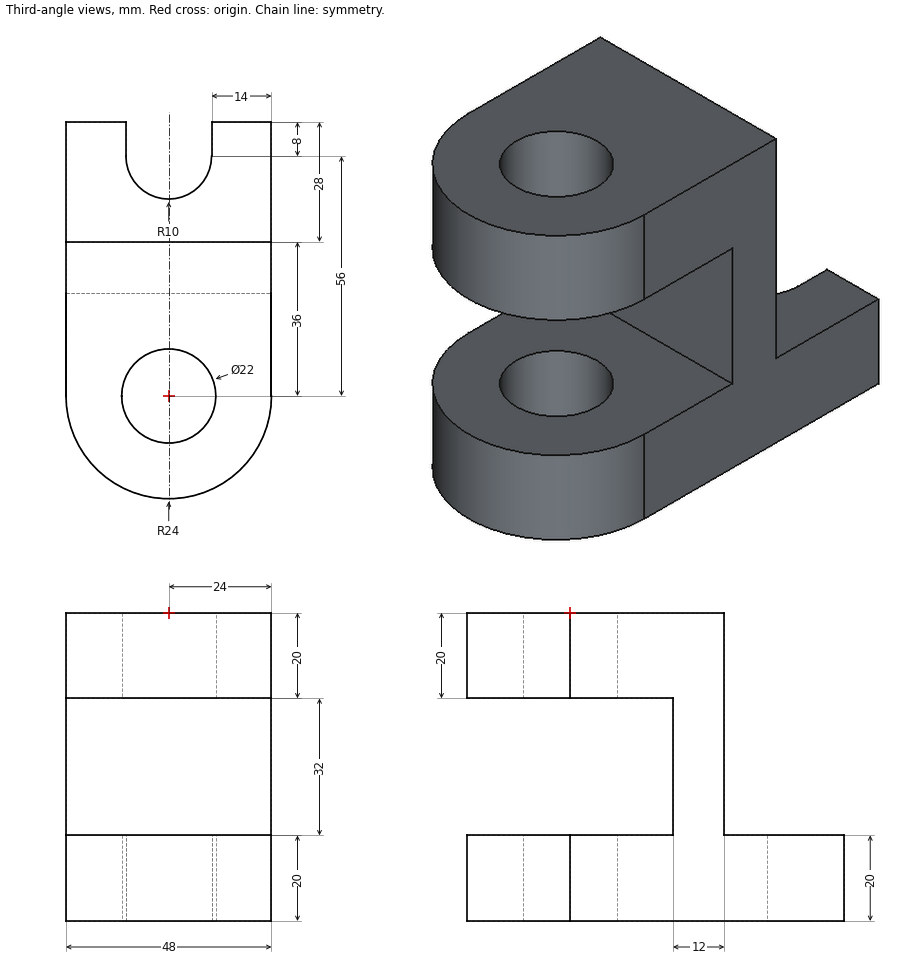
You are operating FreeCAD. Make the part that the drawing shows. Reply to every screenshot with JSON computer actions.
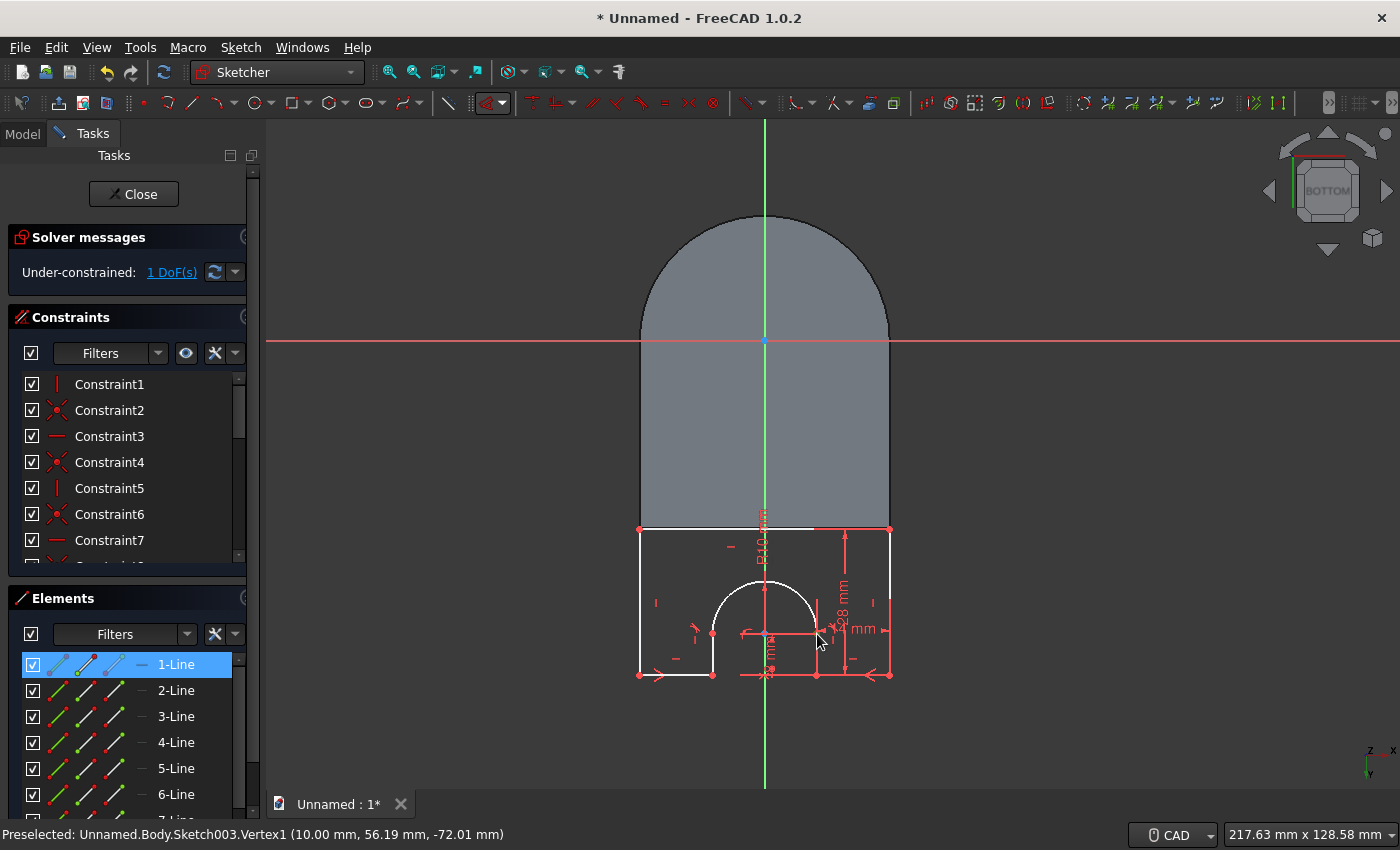
{"action": "key", "text": "i"}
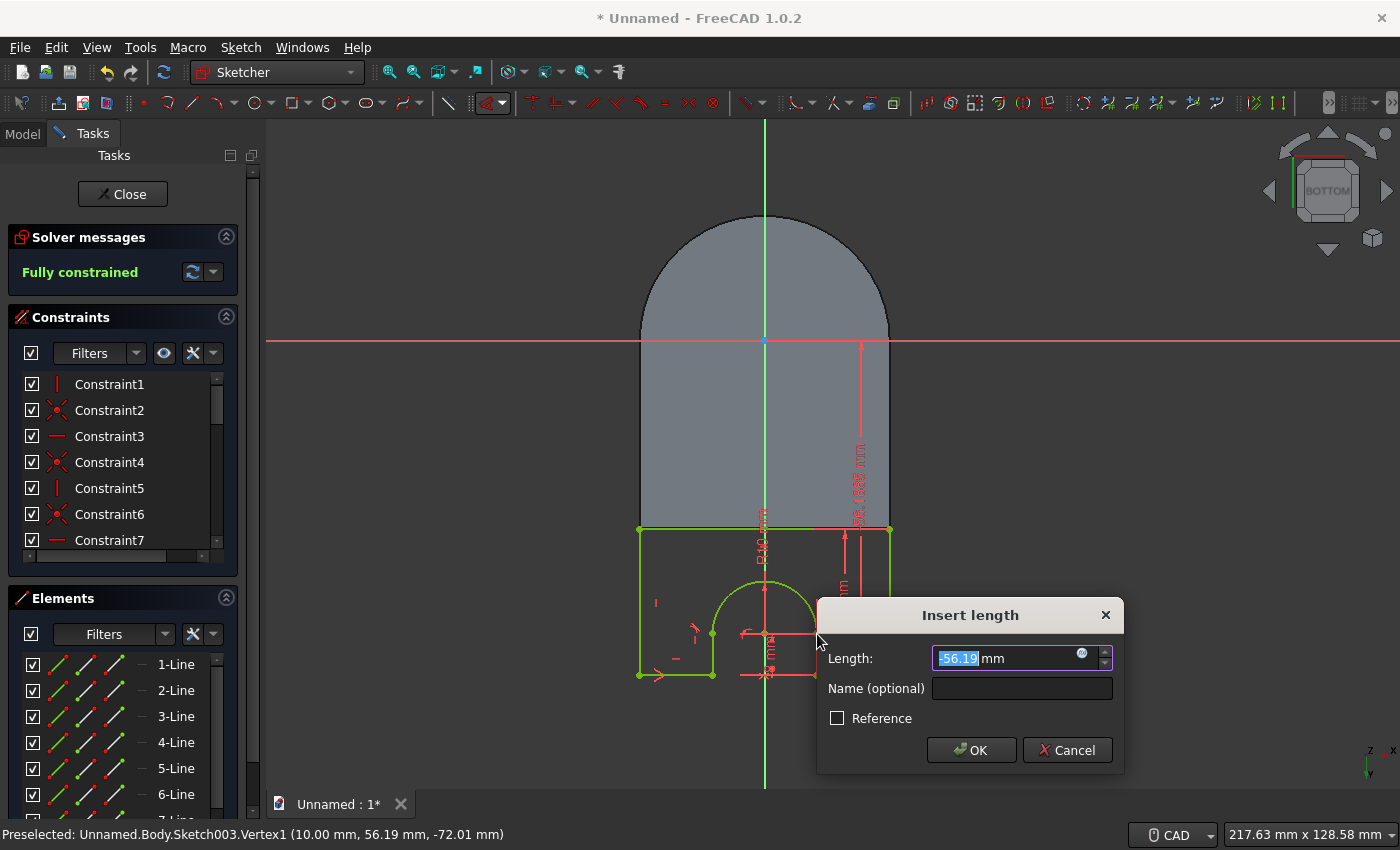
{"action": "type", "text": "-56"}
{"action": "key", "text": "Return"}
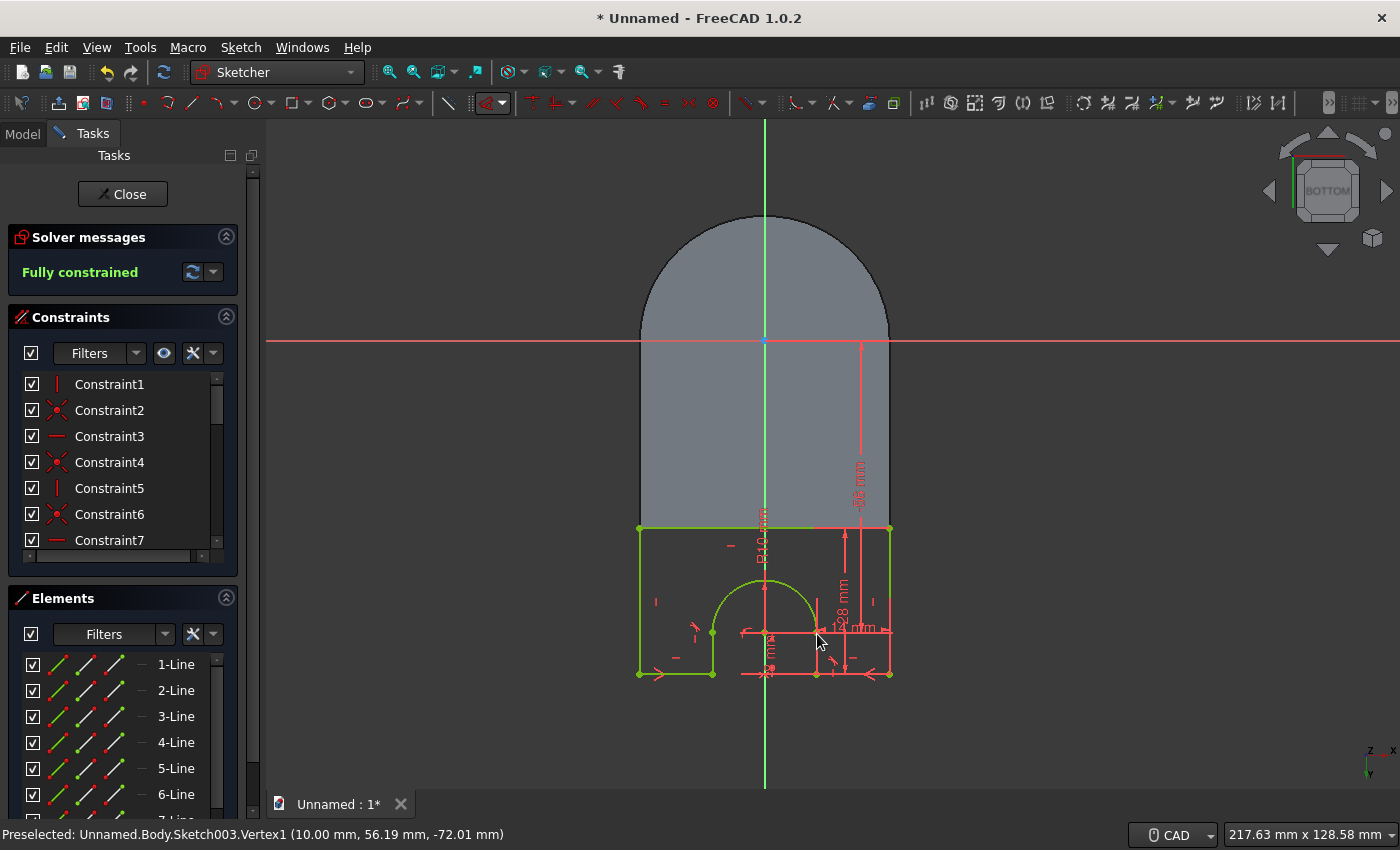
{"action": "left_click", "coordinate": [123, 194]}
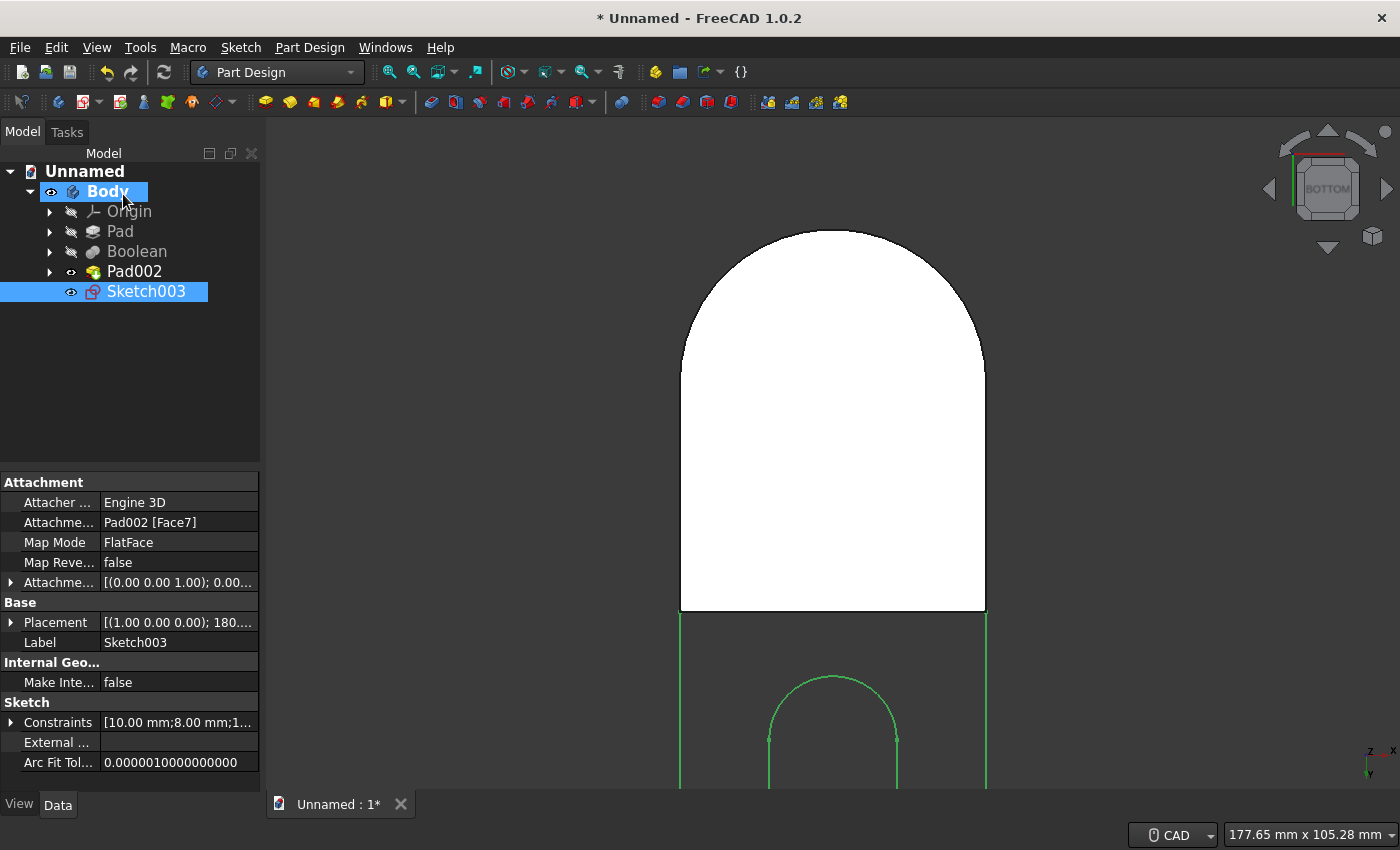
{"action": "left_click", "coordinate": [266, 102]}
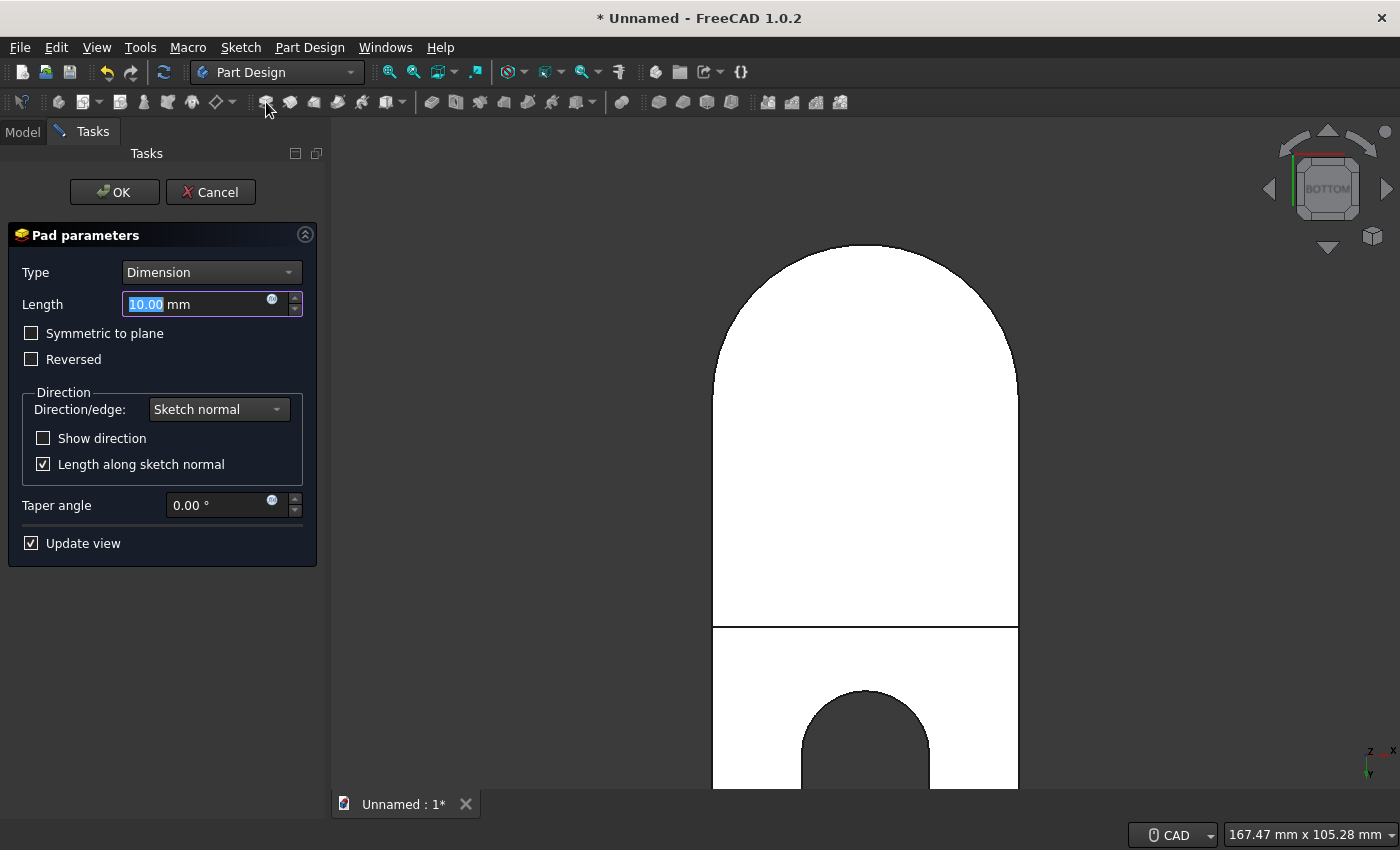
{"action": "type", "text": "20"}
{"action": "key", "text": "Tab"}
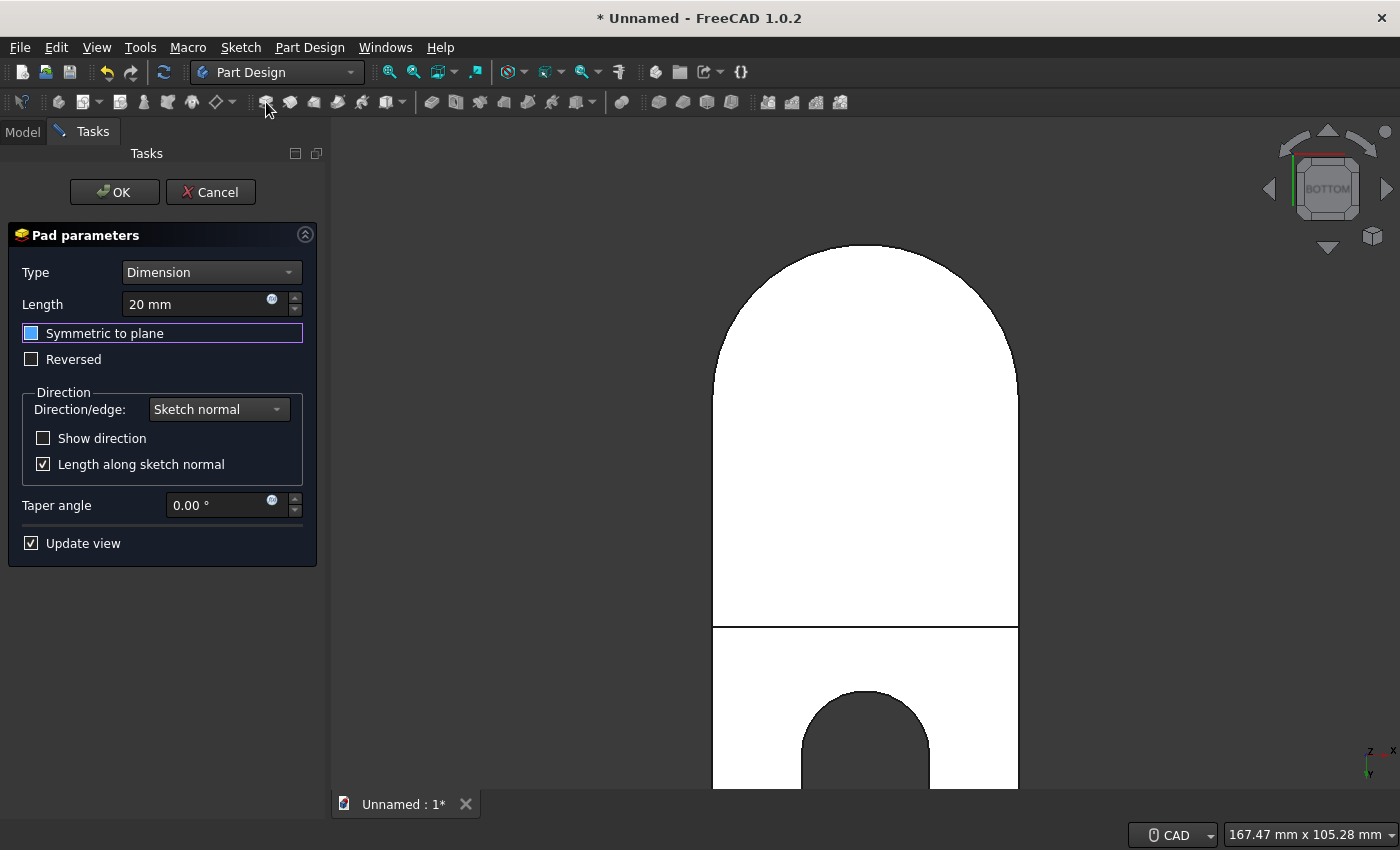
{"action": "left_click", "coordinate": [30, 359]}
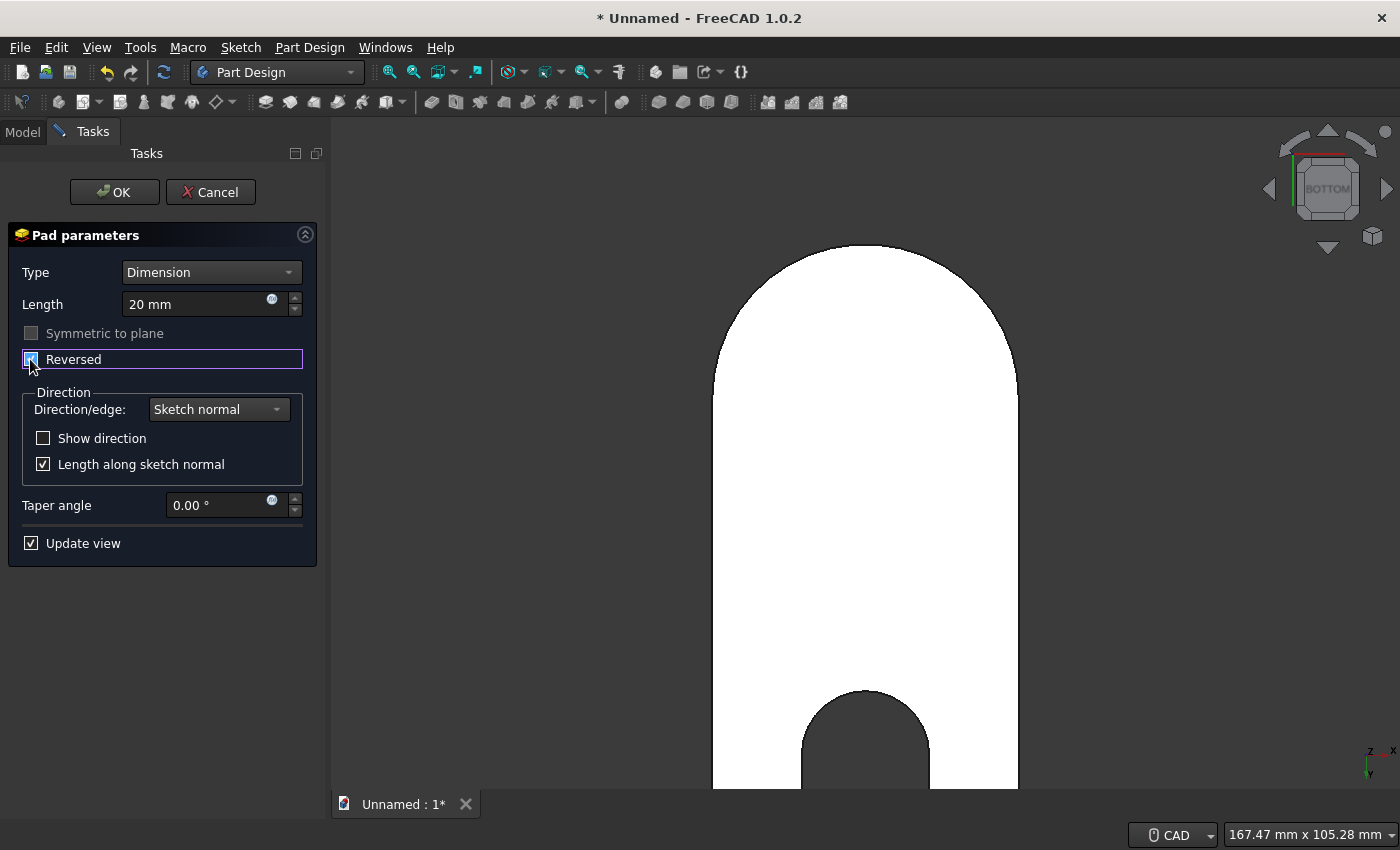
{"action": "left_click", "coordinate": [115, 192]}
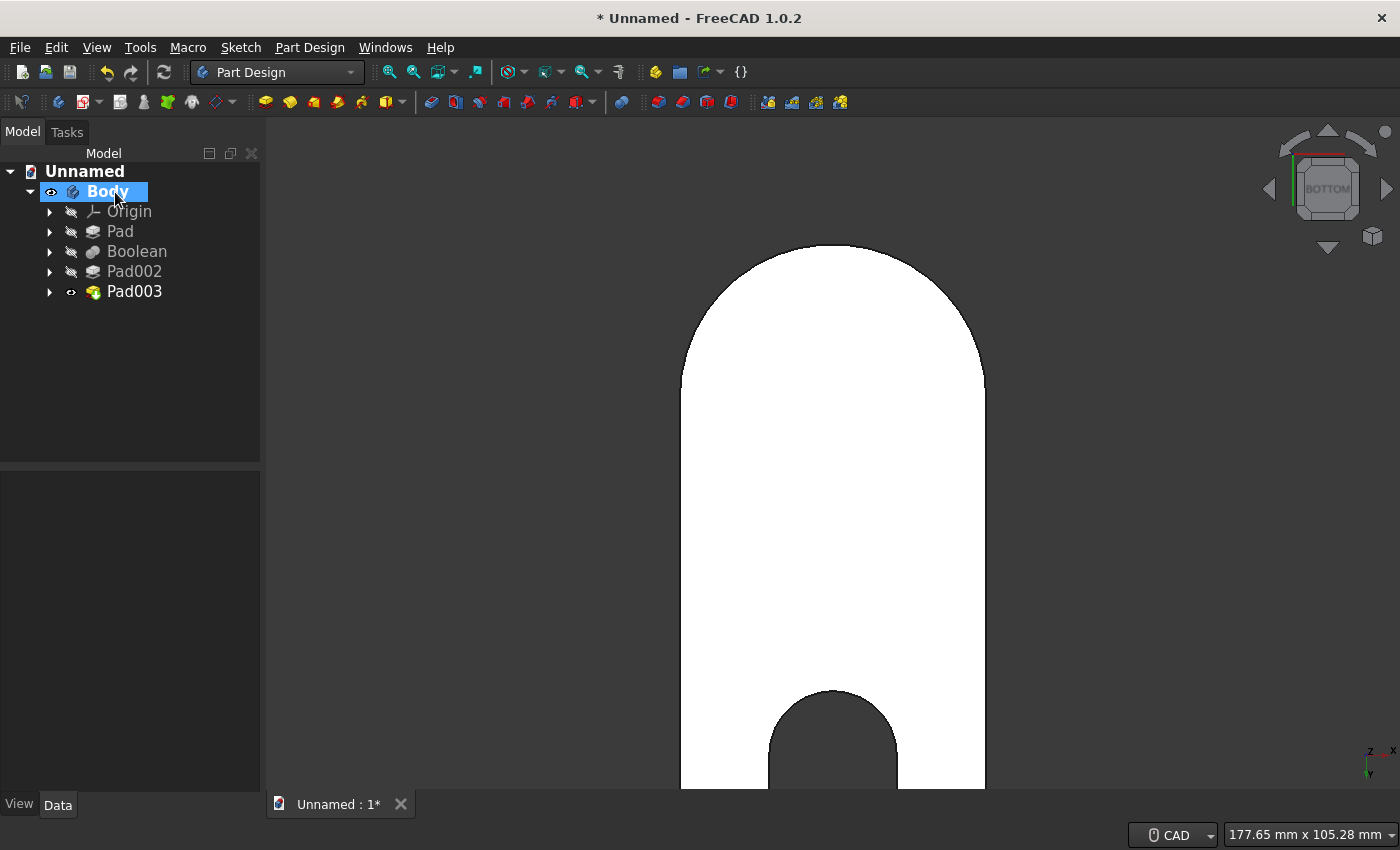
{"action": "key", "text": "v f"}